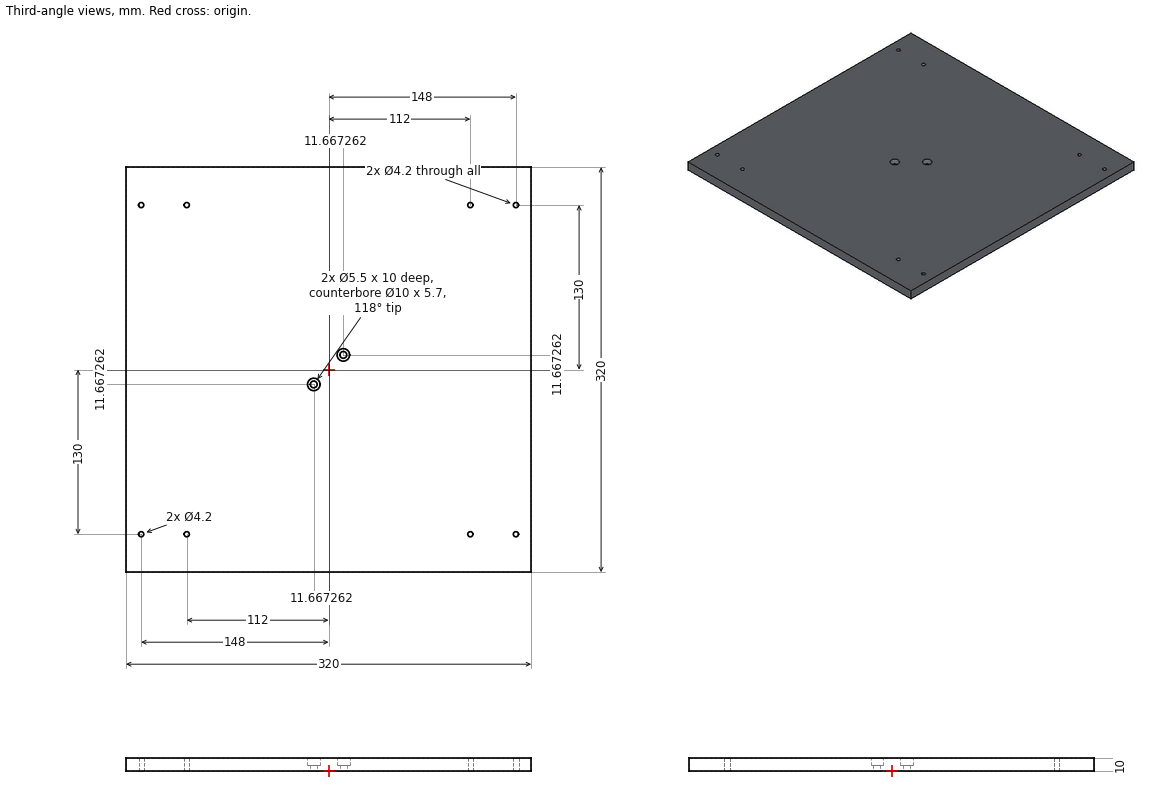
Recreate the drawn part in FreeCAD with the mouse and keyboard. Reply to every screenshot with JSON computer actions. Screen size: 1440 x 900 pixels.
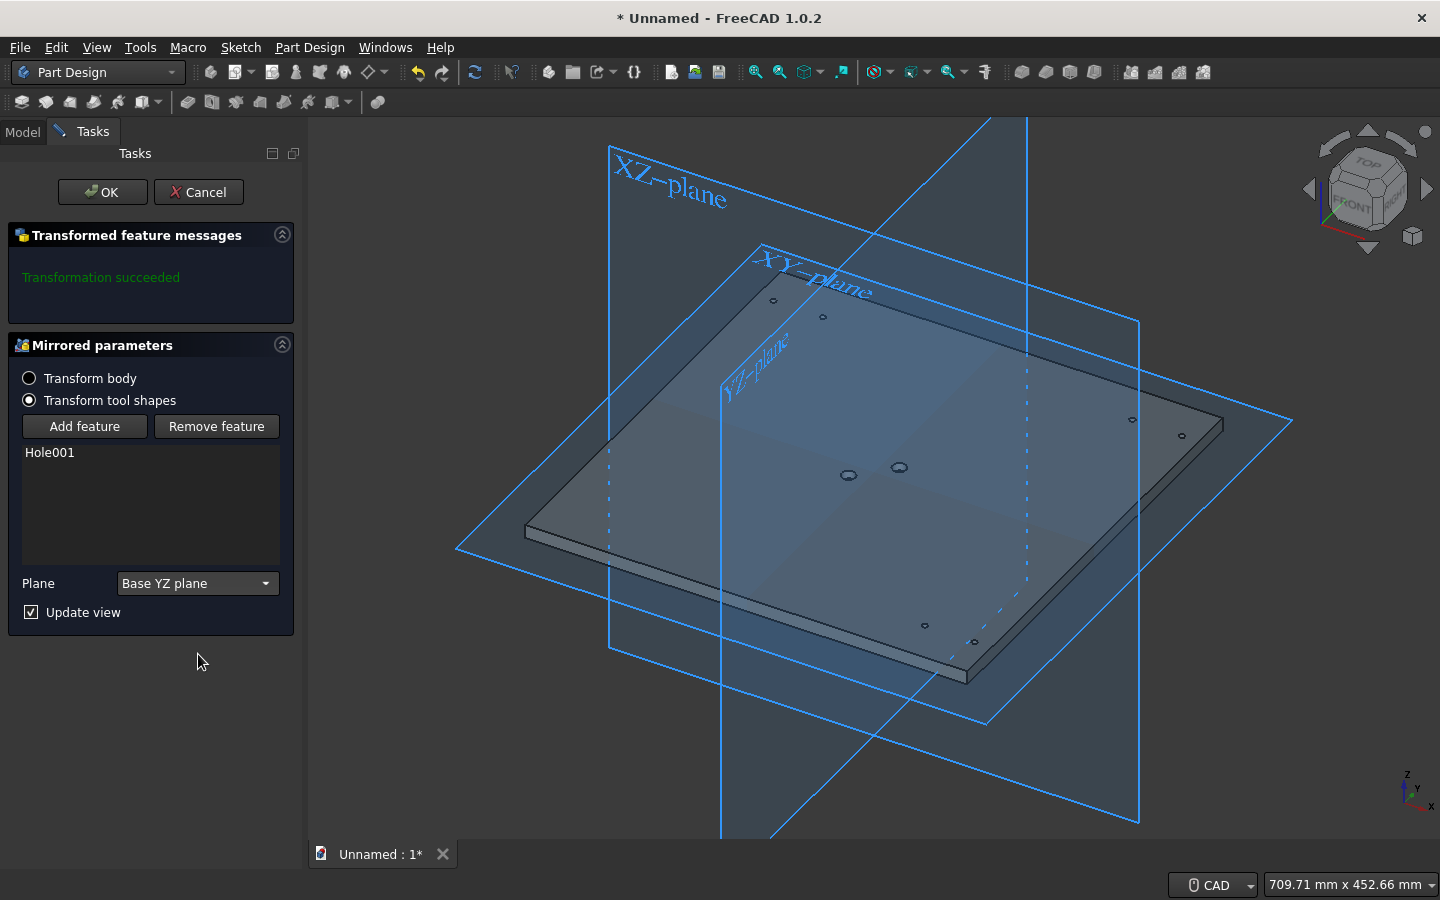
{"action": "left_click", "coordinate": [103, 192]}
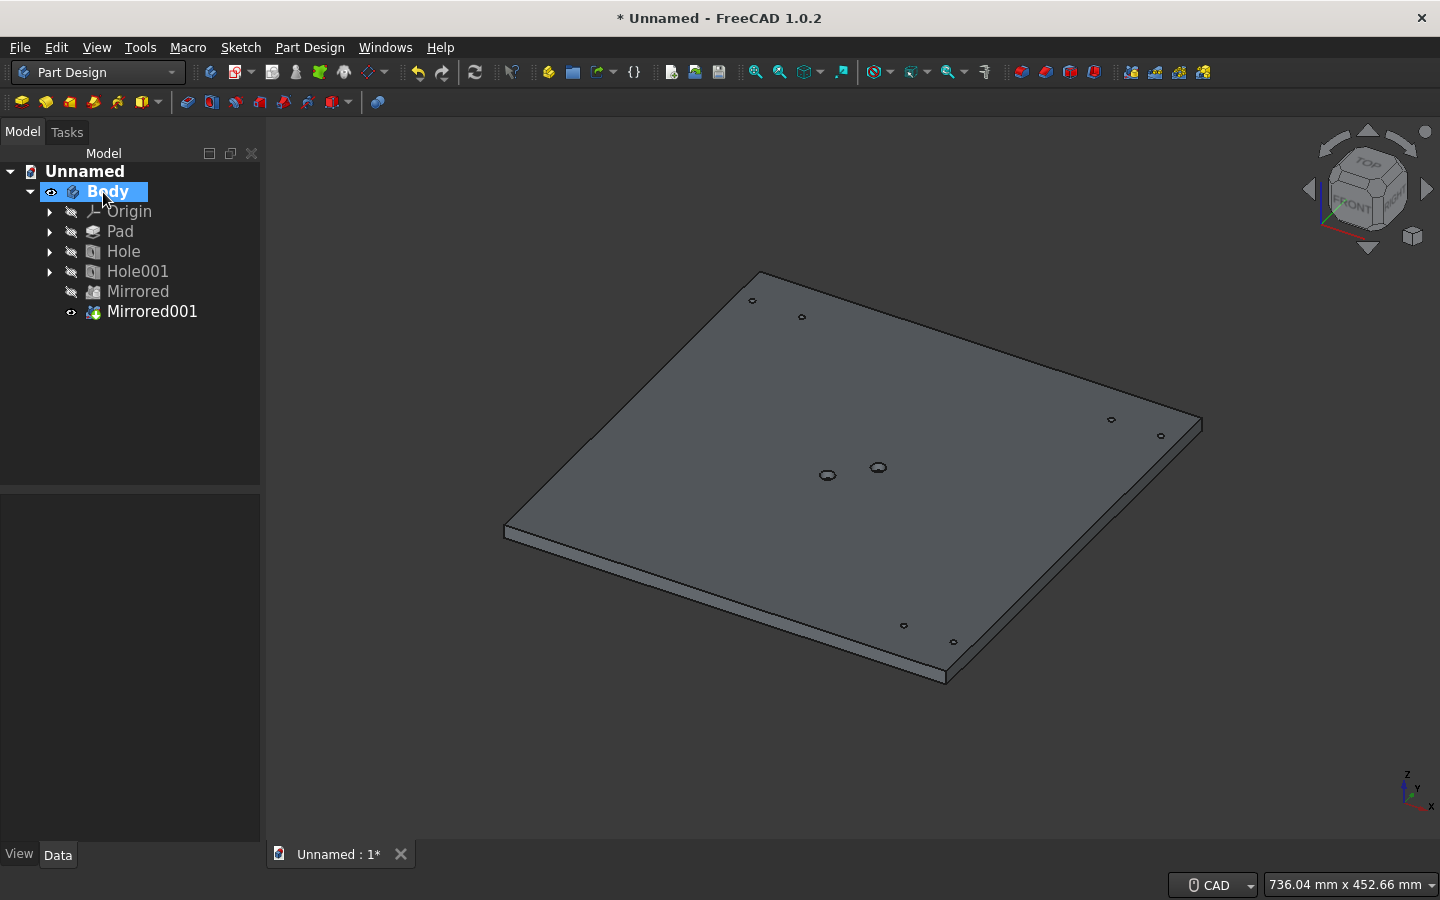
{"action": "key", "text": "5"}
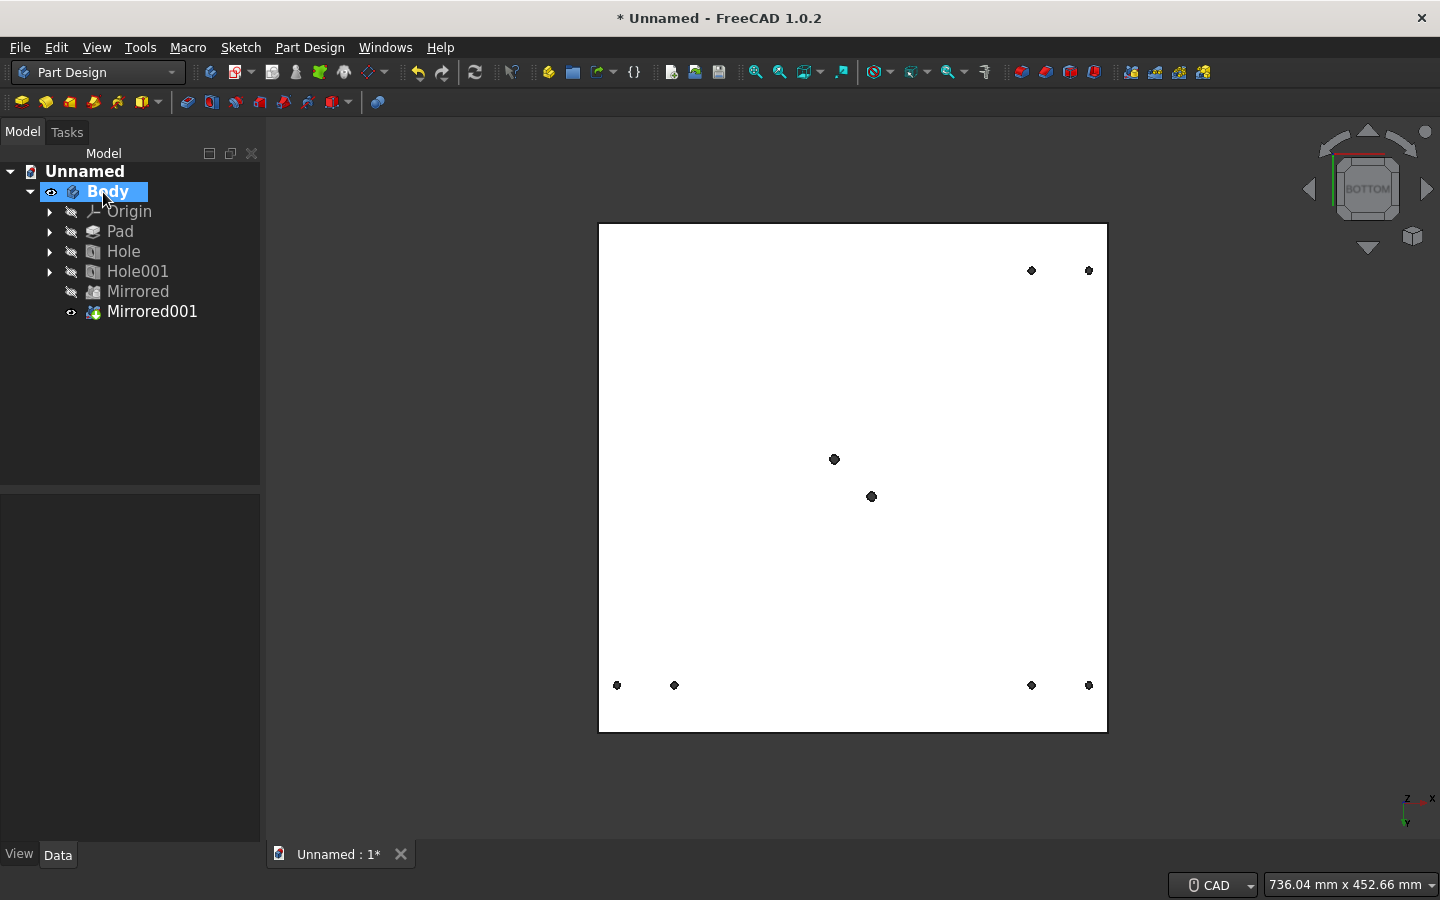
{"action": "left_click", "coordinate": [999, 550]}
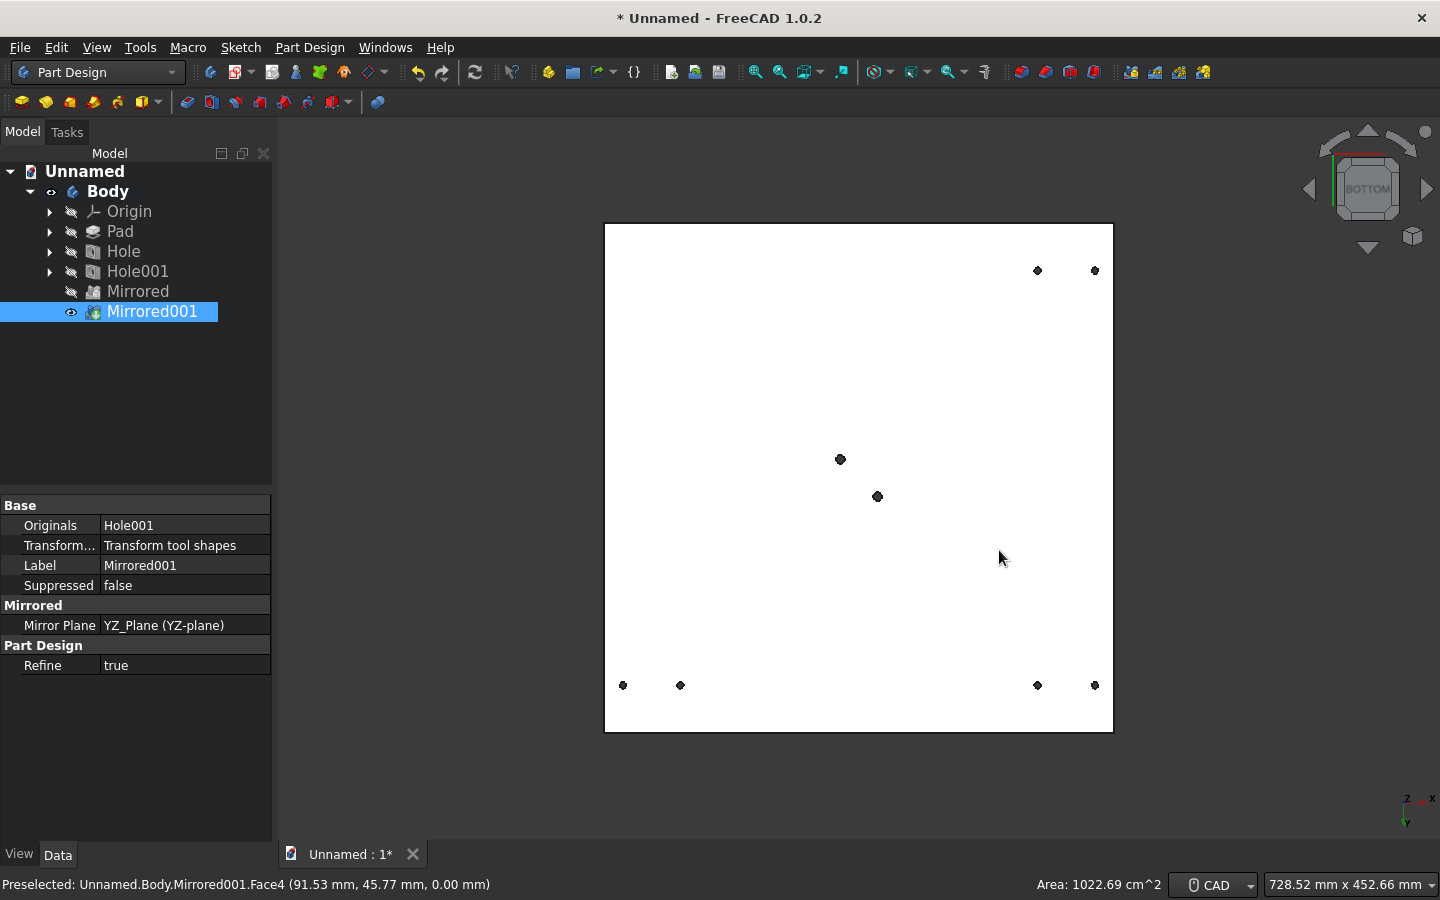
{"action": "left_click", "coordinate": [236, 72]}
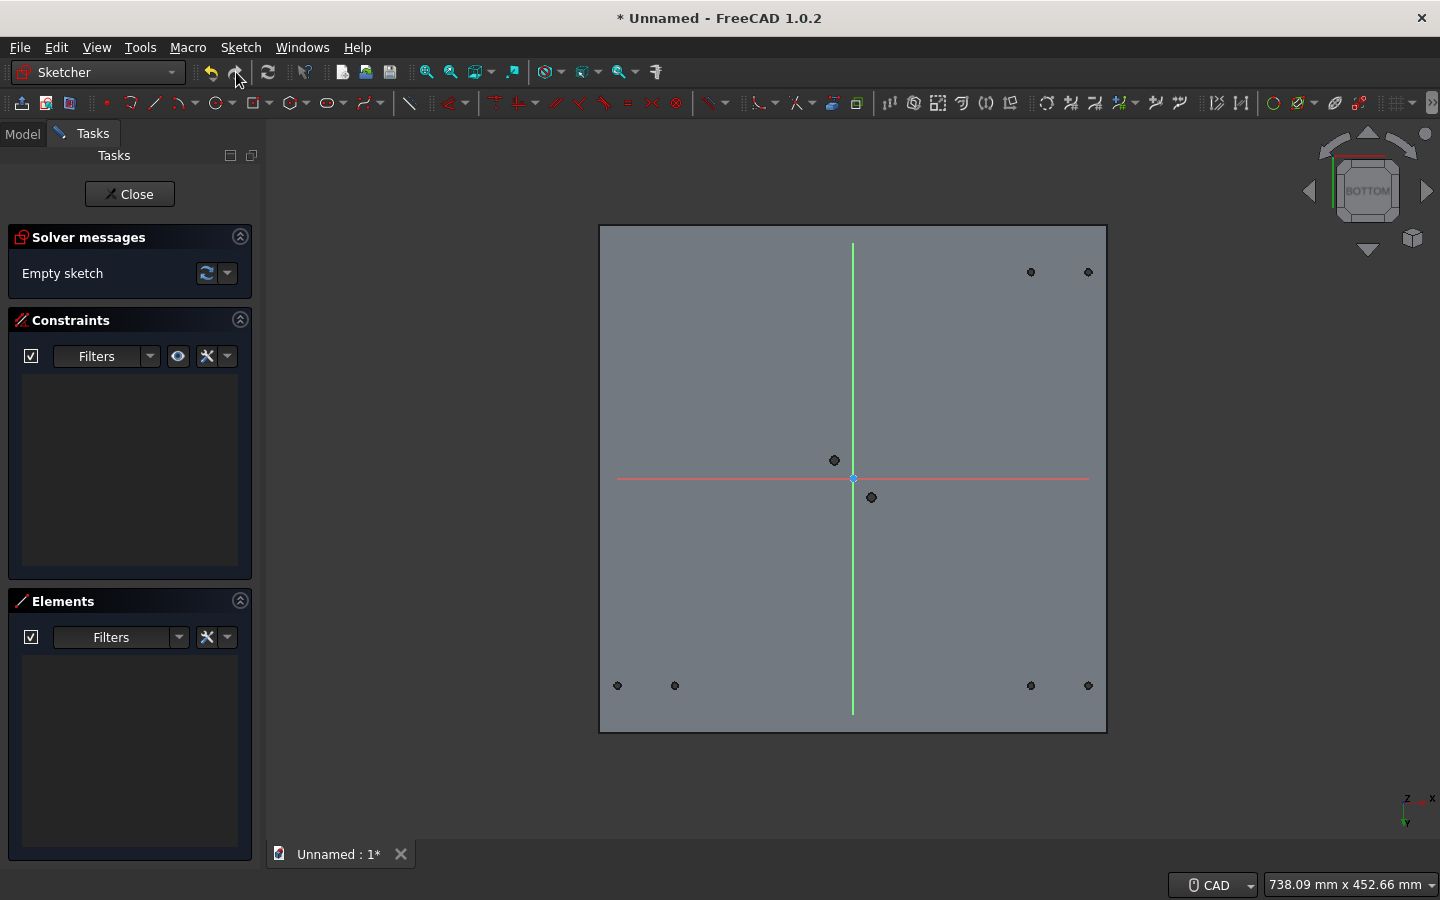
{"action": "scroll", "coordinate": [632, 252], "scroll_direction": "up", "scroll_amount": 12}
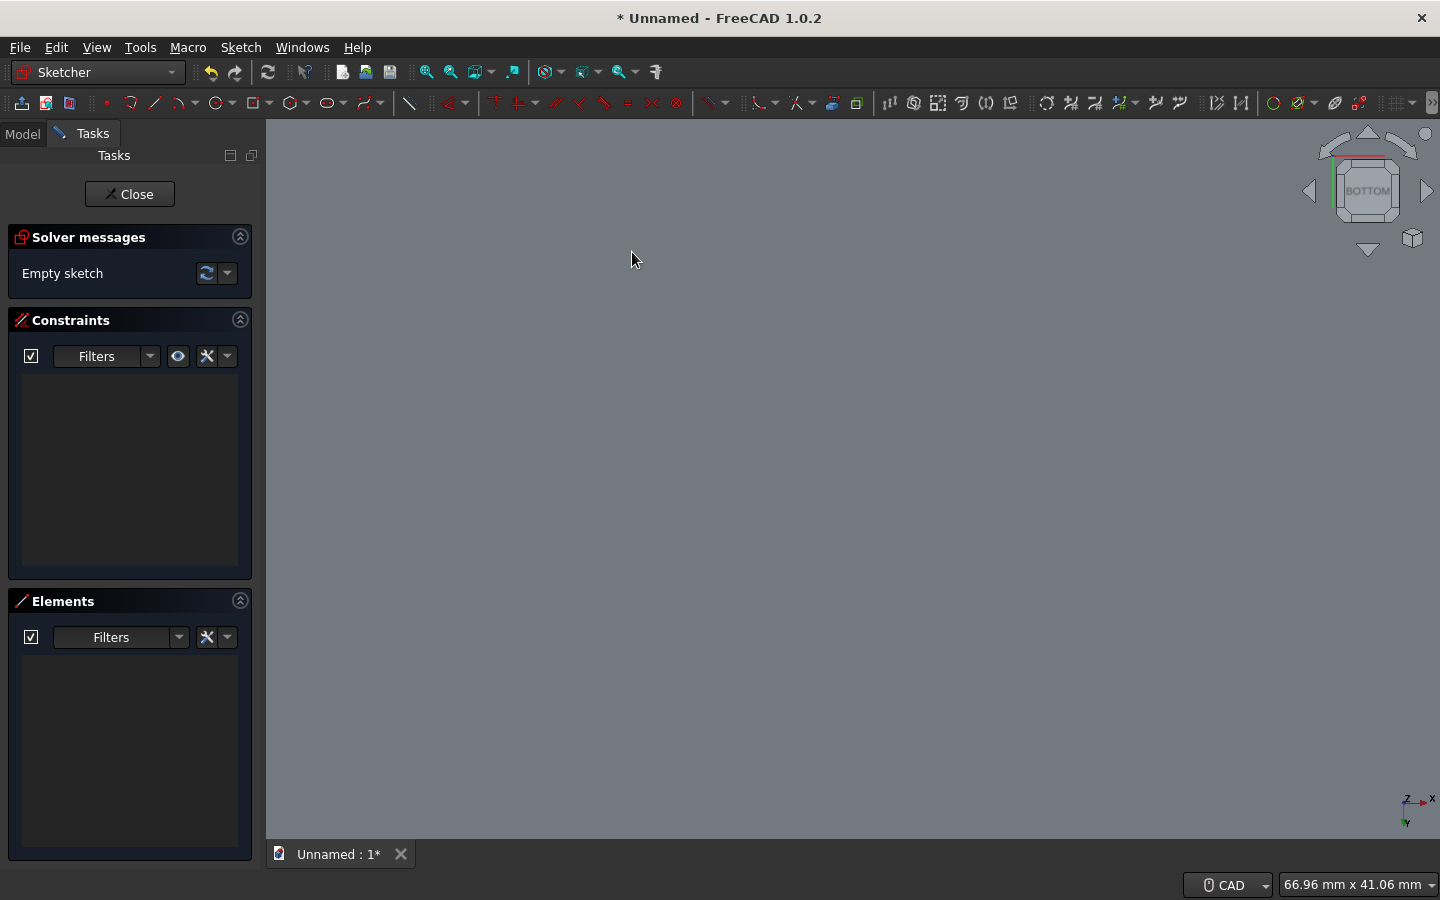
{"action": "key", "text": "g c"}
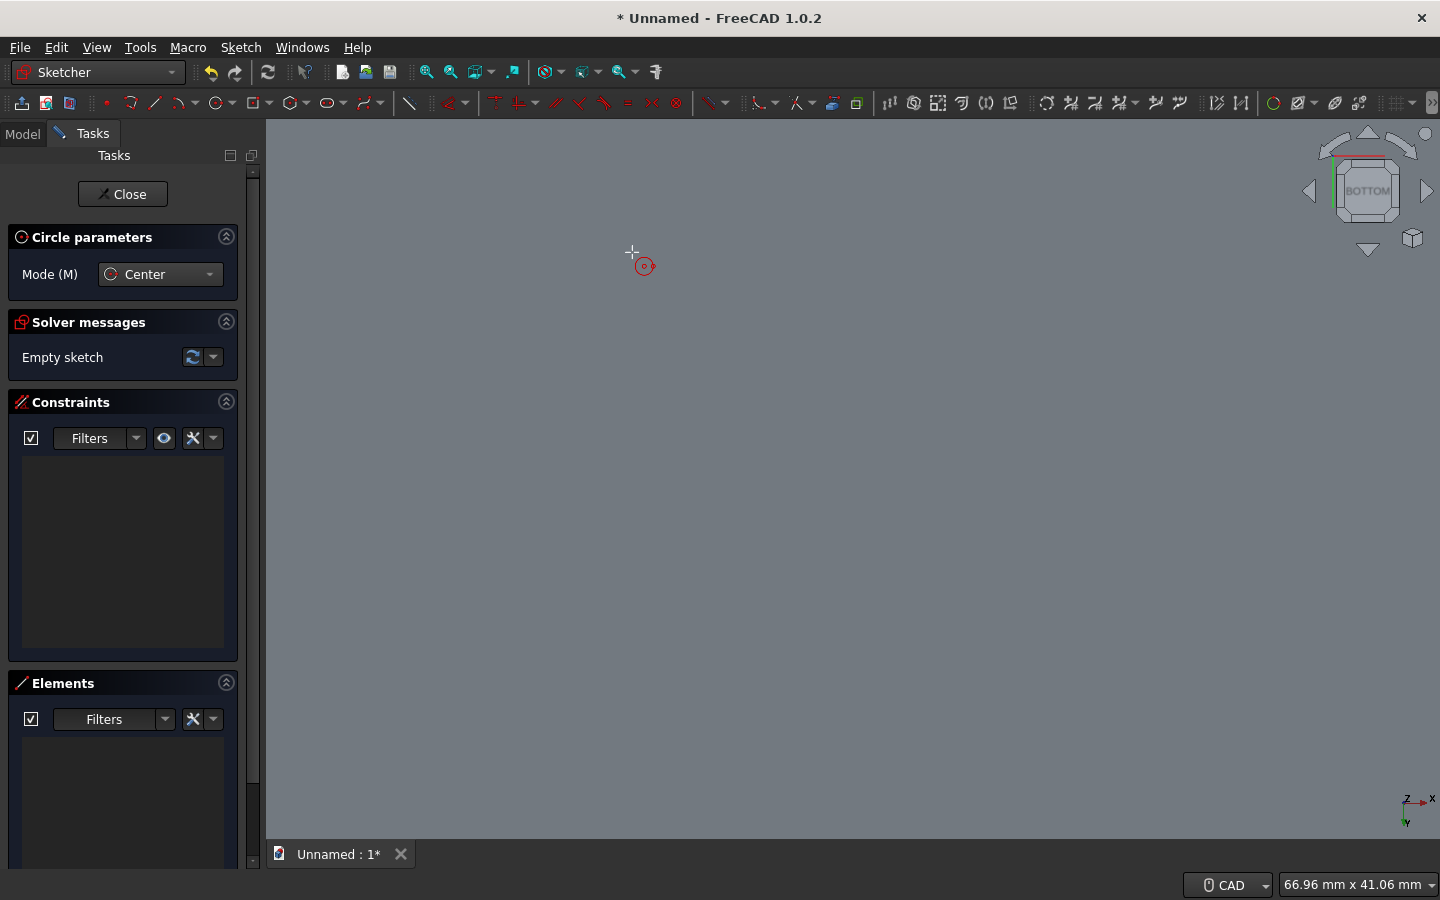
{"action": "left_click", "coordinate": [470, 473]}
{"action": "mouse_move", "coordinate": [496, 447]}